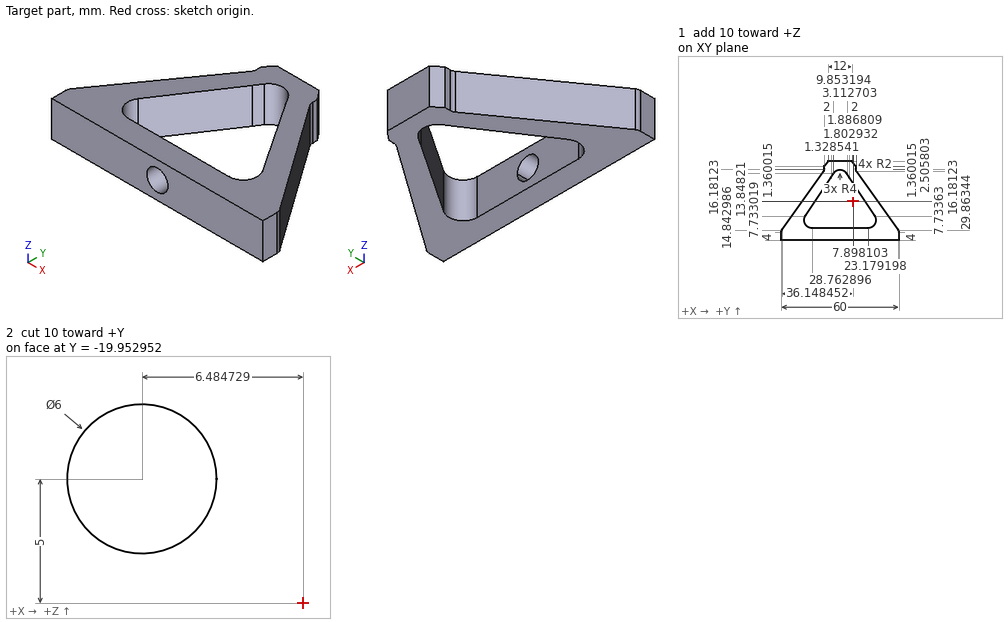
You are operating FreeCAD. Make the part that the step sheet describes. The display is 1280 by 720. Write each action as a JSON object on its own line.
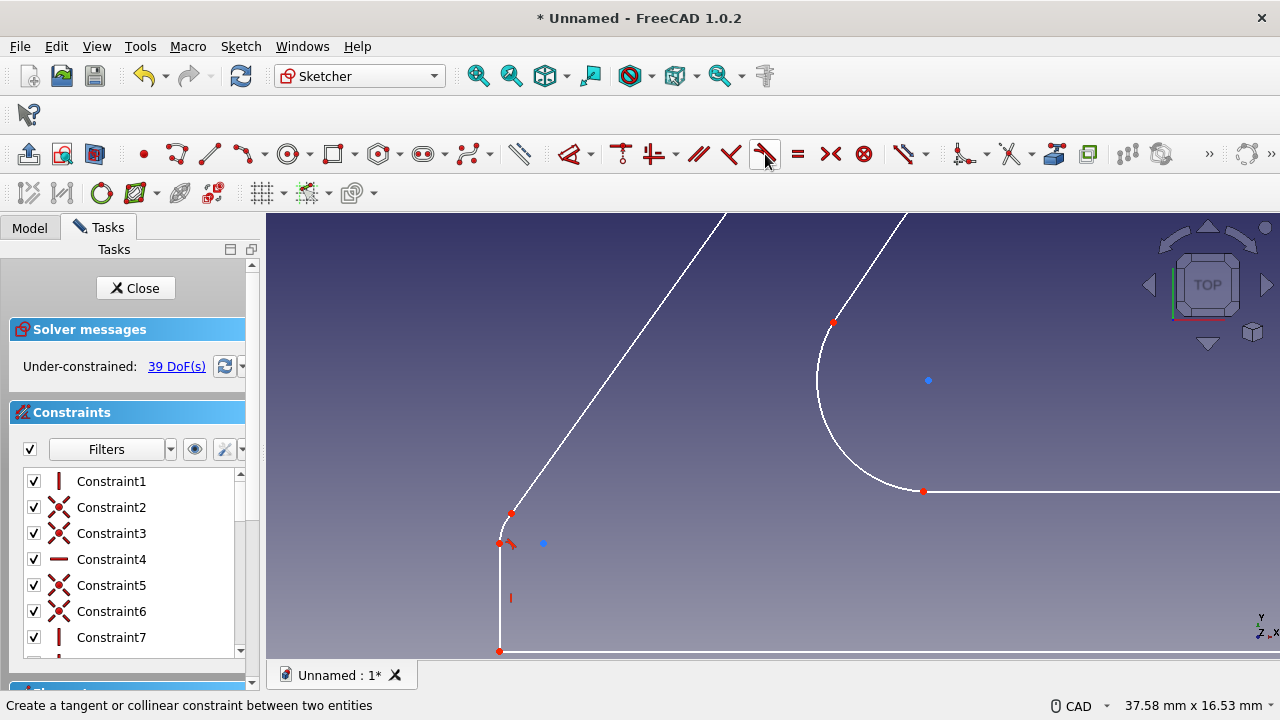
{"action": "scroll", "coordinate": [506, 543], "scroll_direction": "down", "scroll_amount": 7}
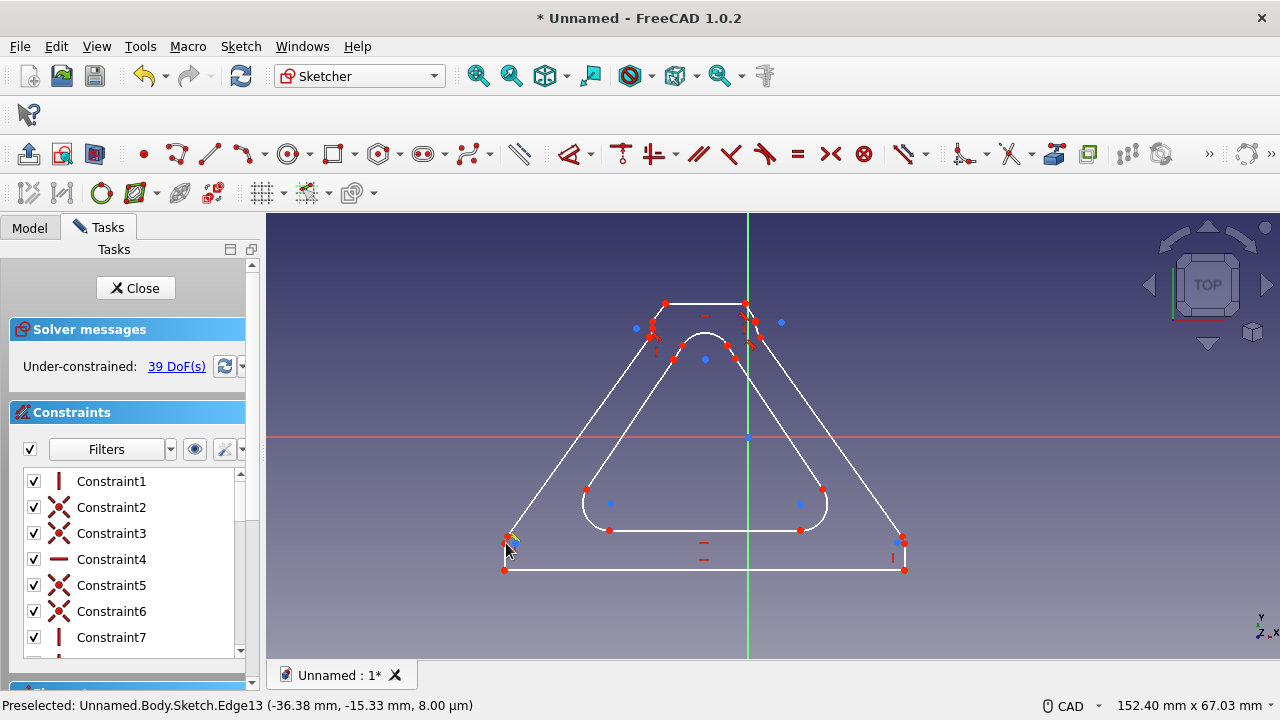
{"action": "scroll", "coordinate": [905, 562], "scroll_direction": "up", "scroll_amount": 3}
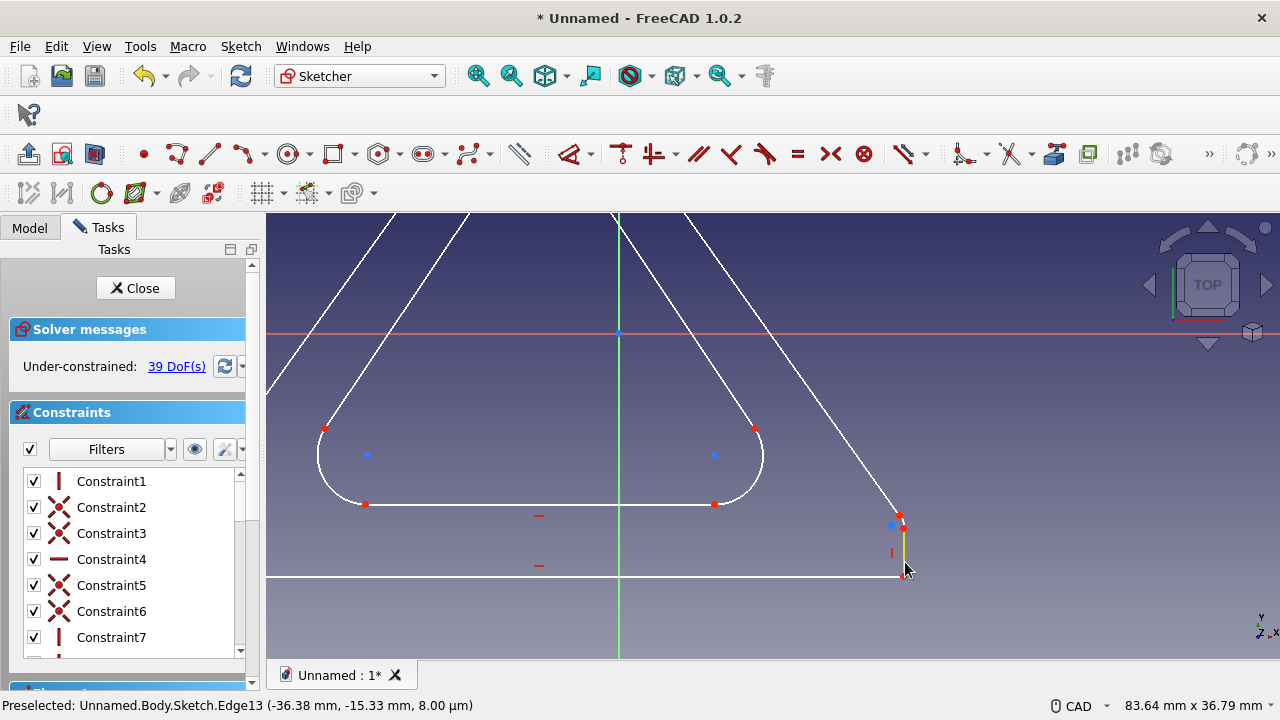
{"action": "left_click", "coordinate": [904, 562]}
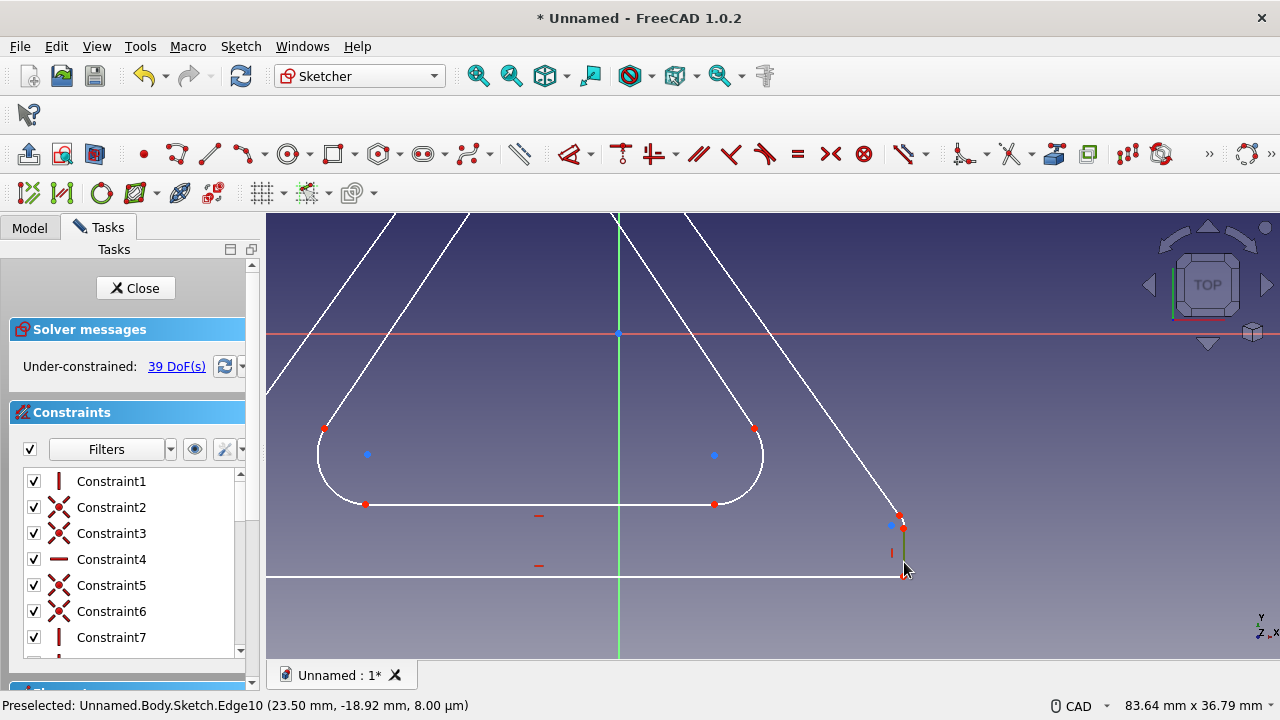
{"action": "scroll", "coordinate": [903, 521], "scroll_direction": "up", "scroll_amount": 4}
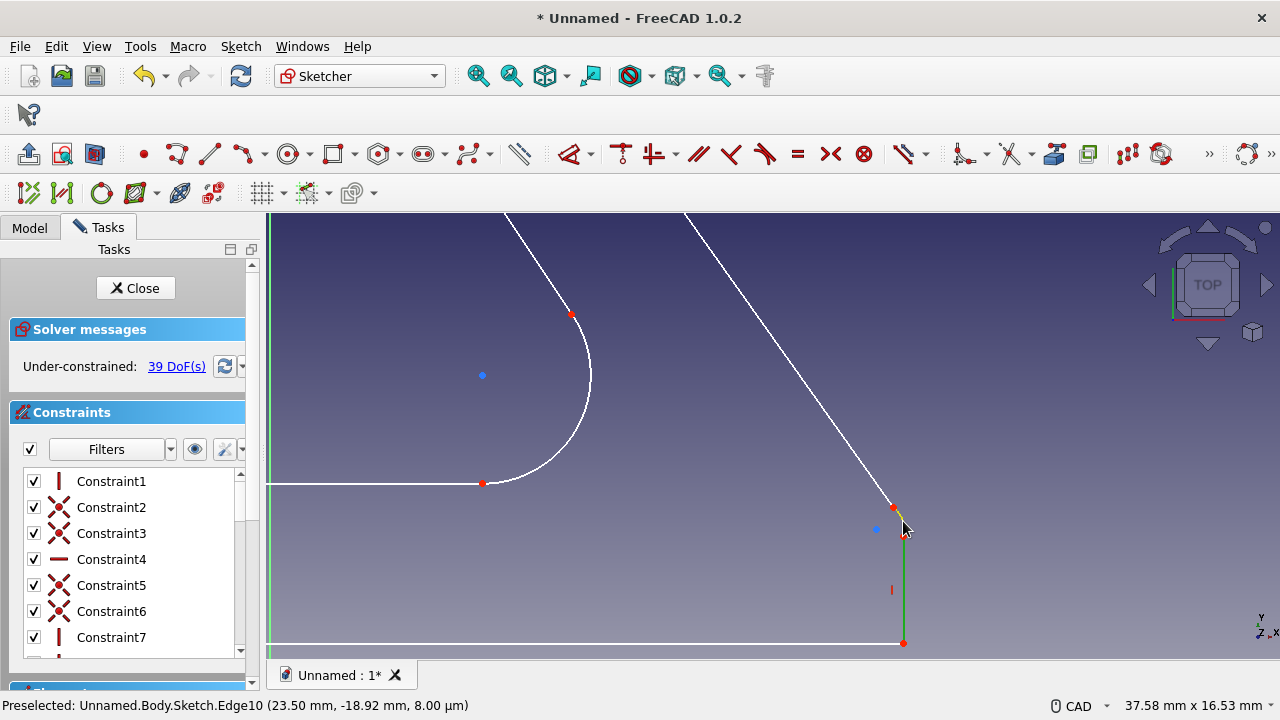
{"action": "left_click", "coordinate": [903, 520]}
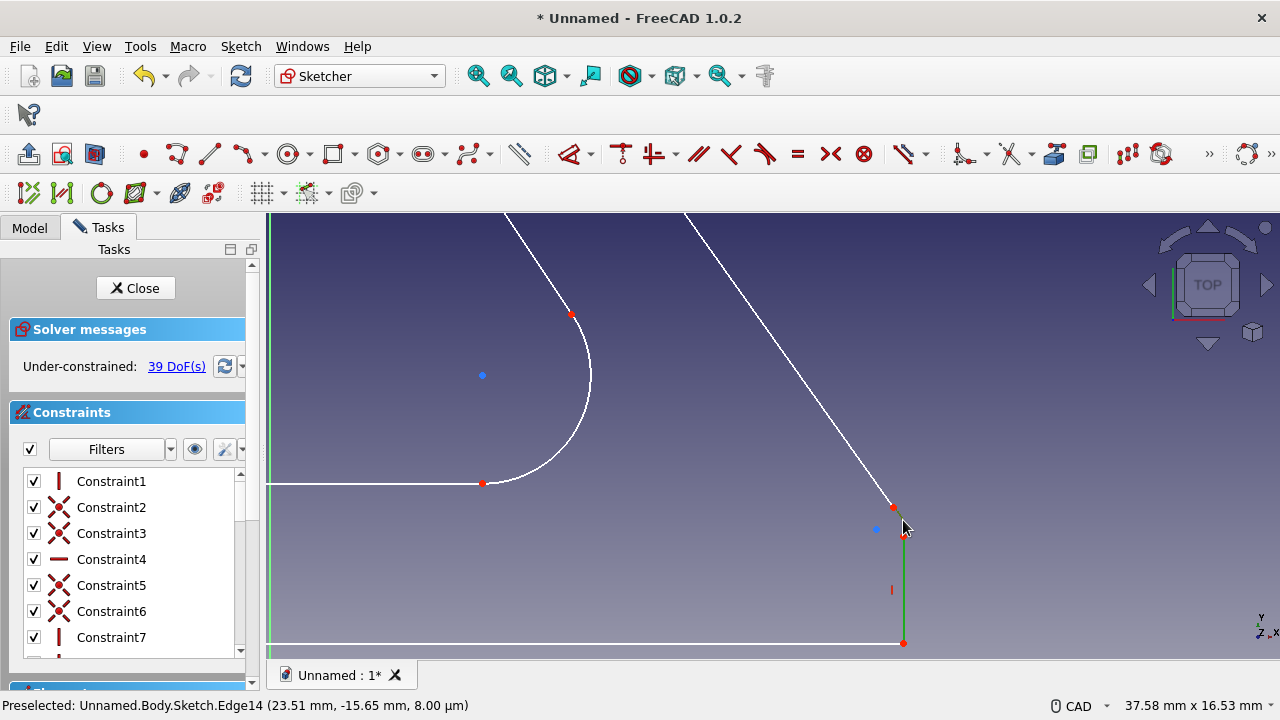
{"action": "left_click", "coordinate": [765, 154]}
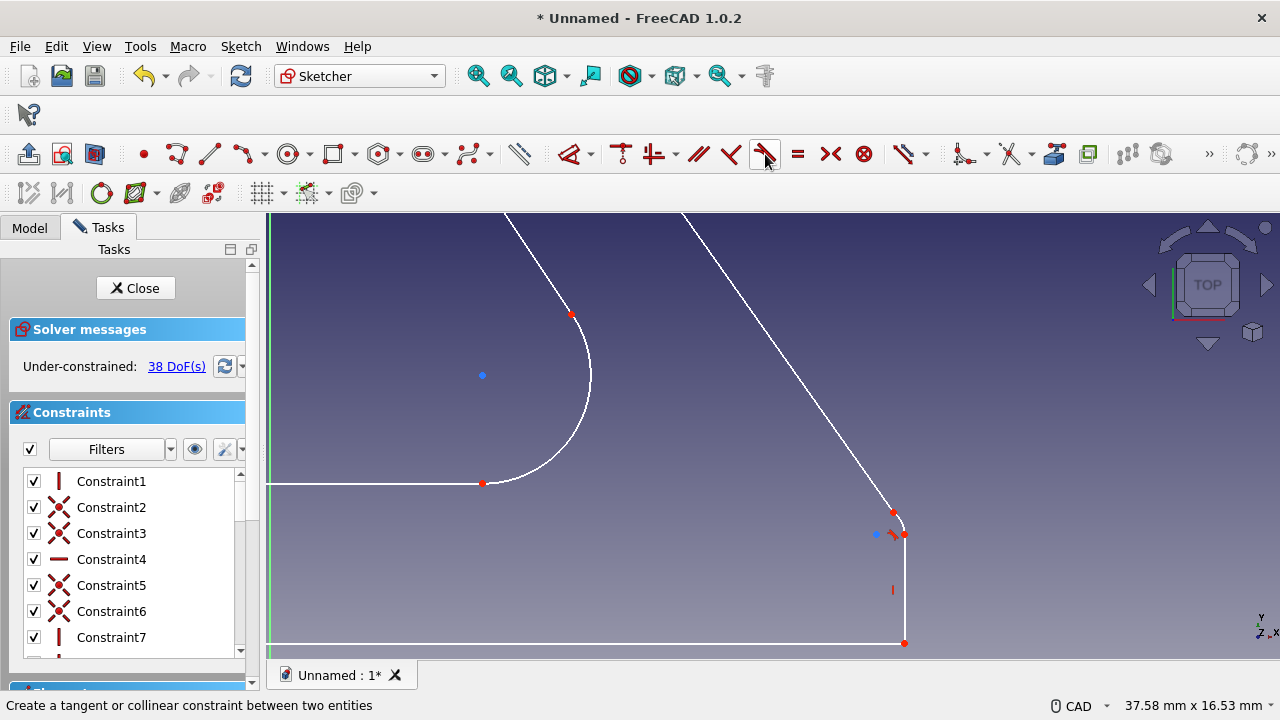
{"action": "scroll", "coordinate": [904, 545], "scroll_direction": "down", "scroll_amount": 7}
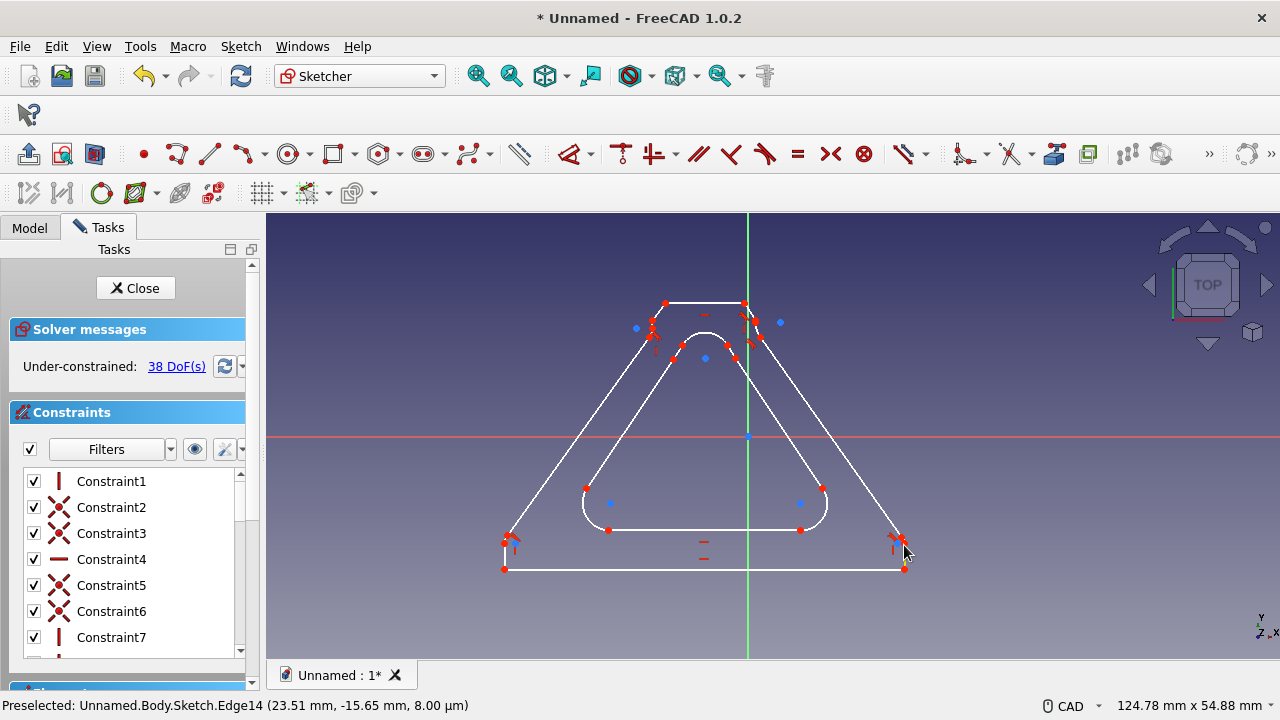
{"action": "left_click", "coordinate": [613, 450]}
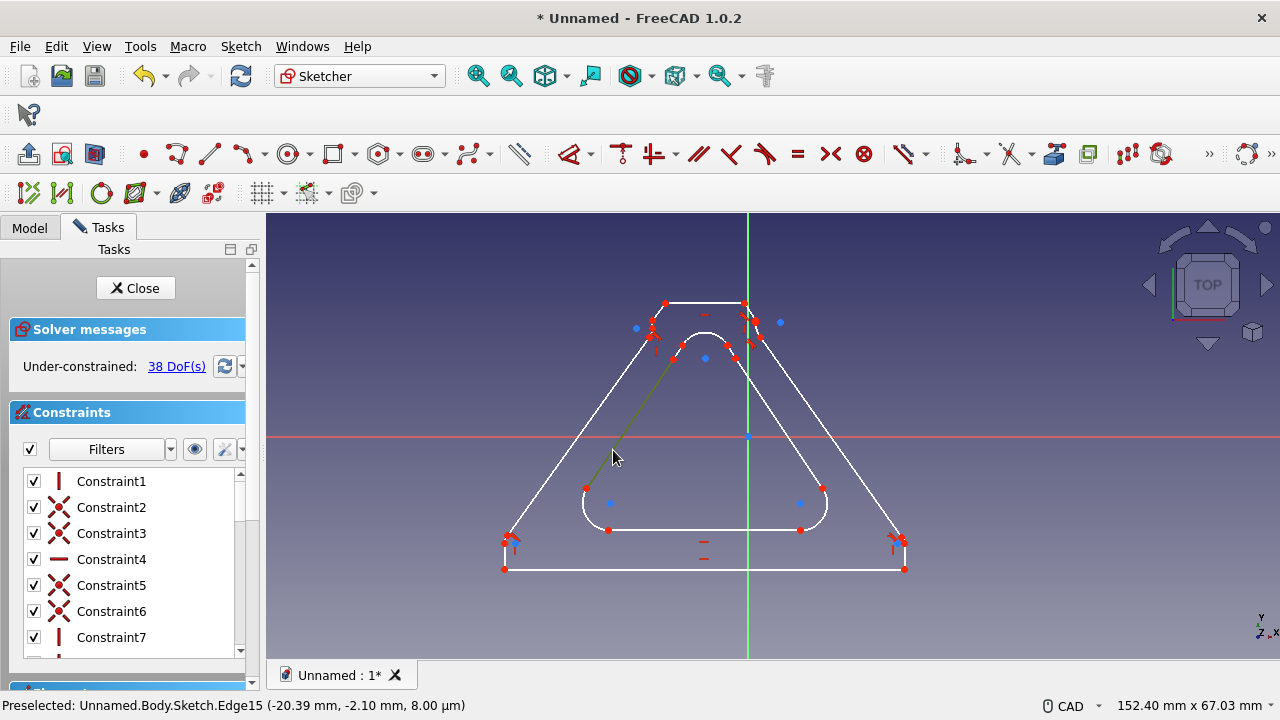
{"action": "left_click", "coordinate": [583, 505]}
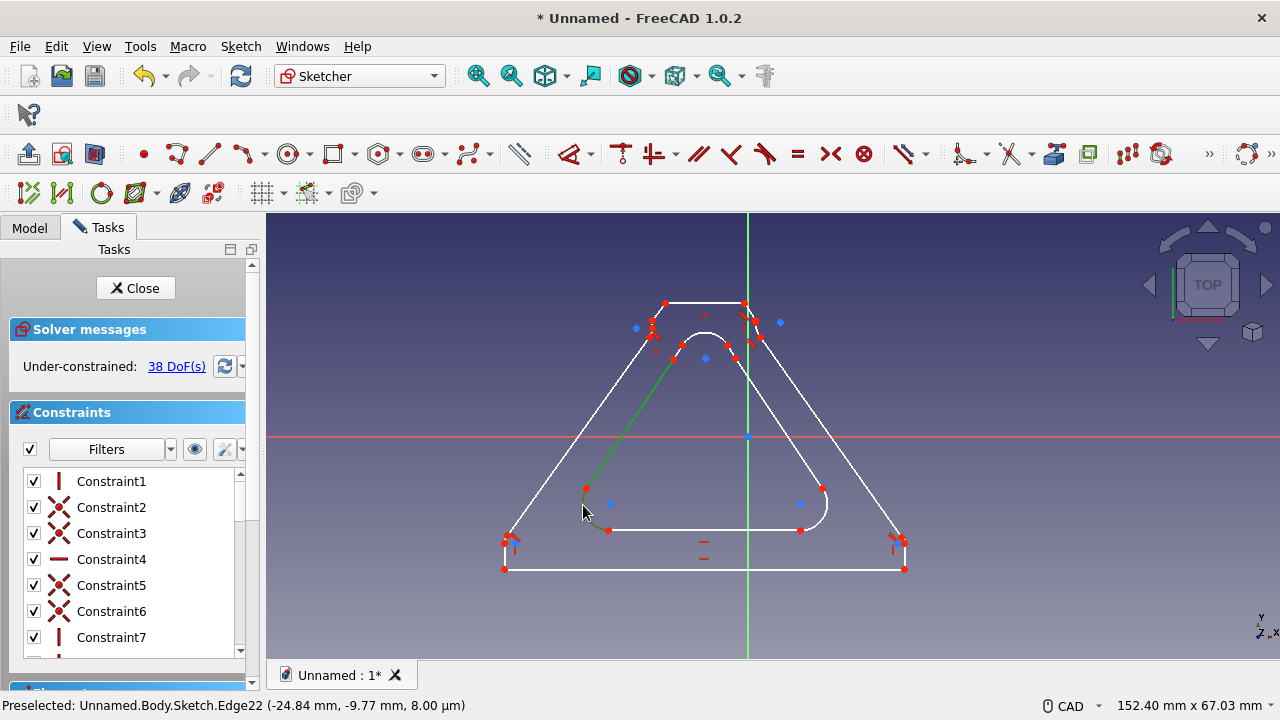
{"action": "left_click", "coordinate": [765, 154]}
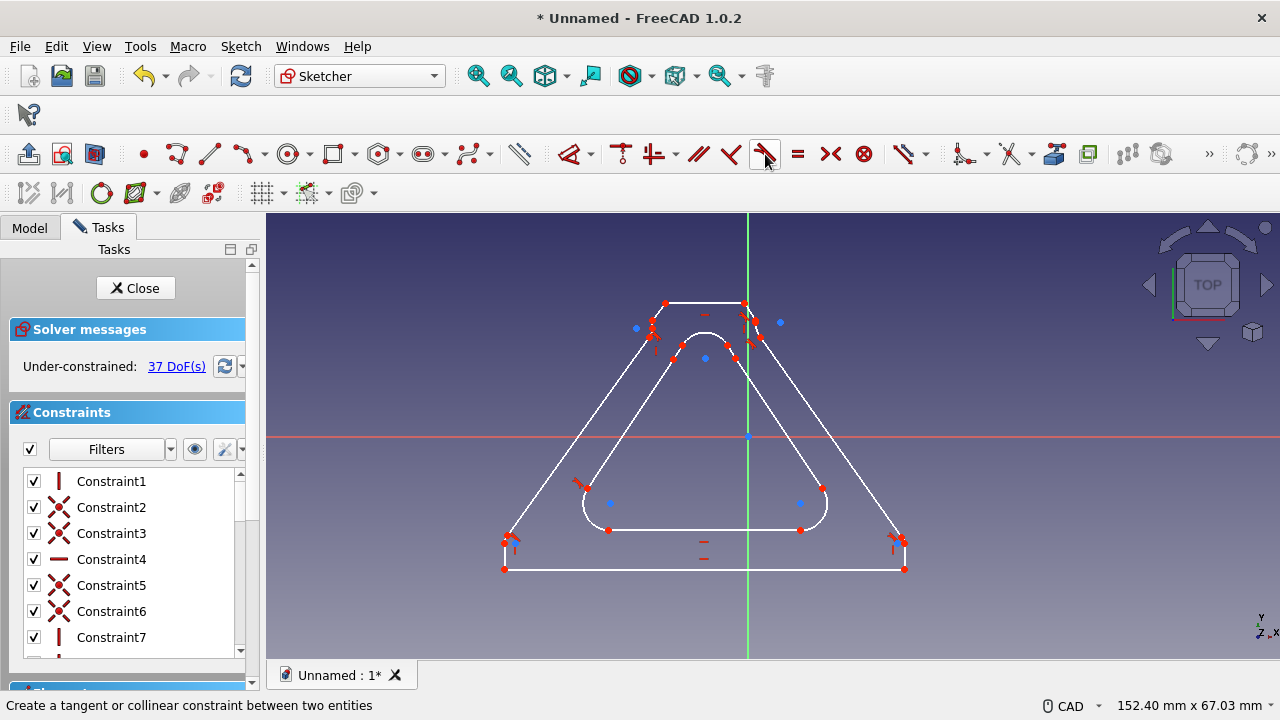
{"action": "scroll", "coordinate": [678, 352], "scroll_direction": "up", "scroll_amount": 3}